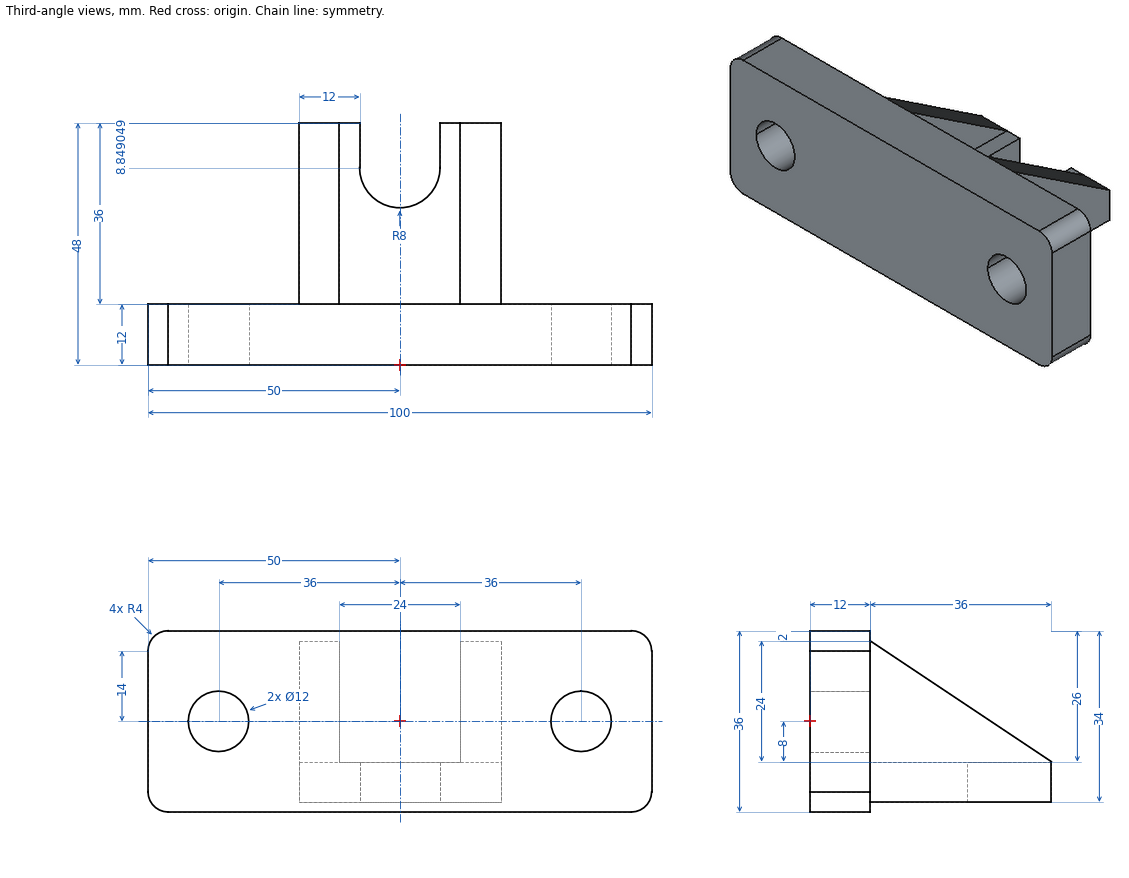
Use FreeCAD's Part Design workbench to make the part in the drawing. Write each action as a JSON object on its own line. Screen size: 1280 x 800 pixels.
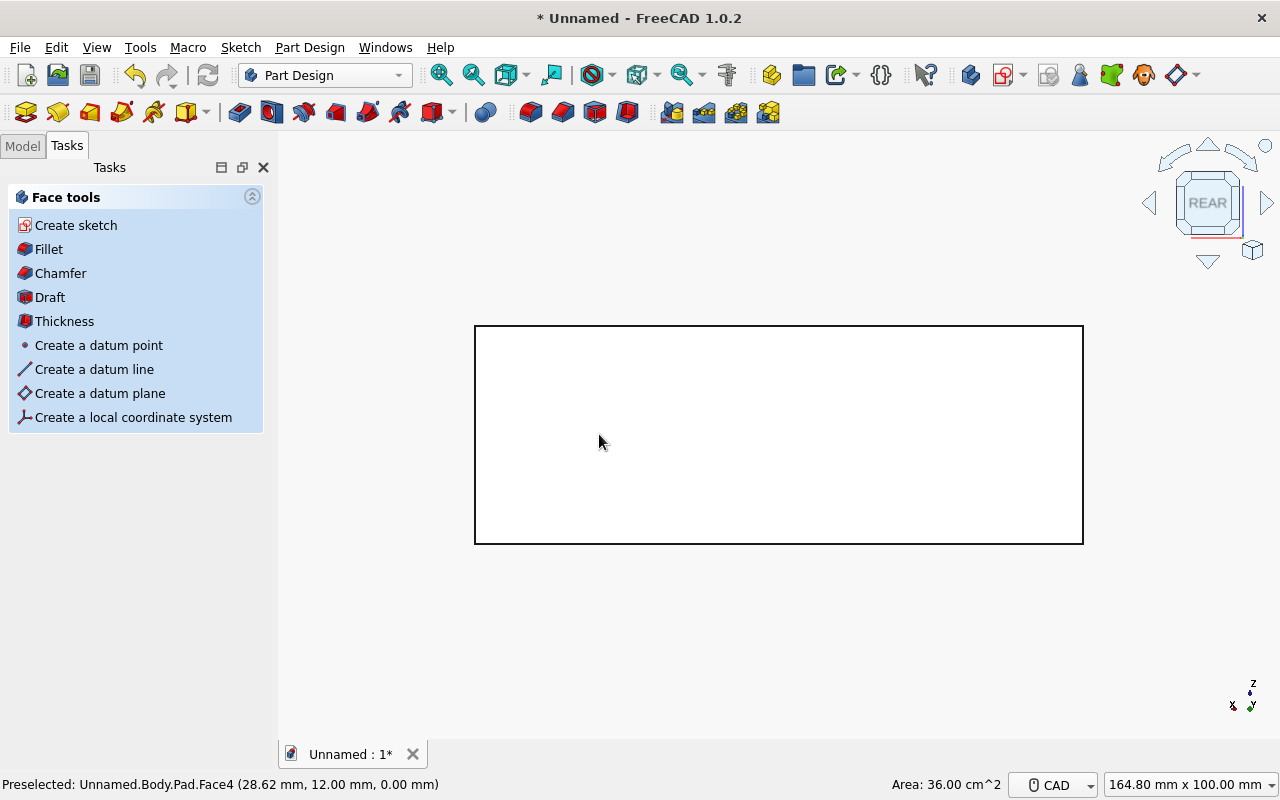
{"action": "left_click", "coordinate": [1004, 76]}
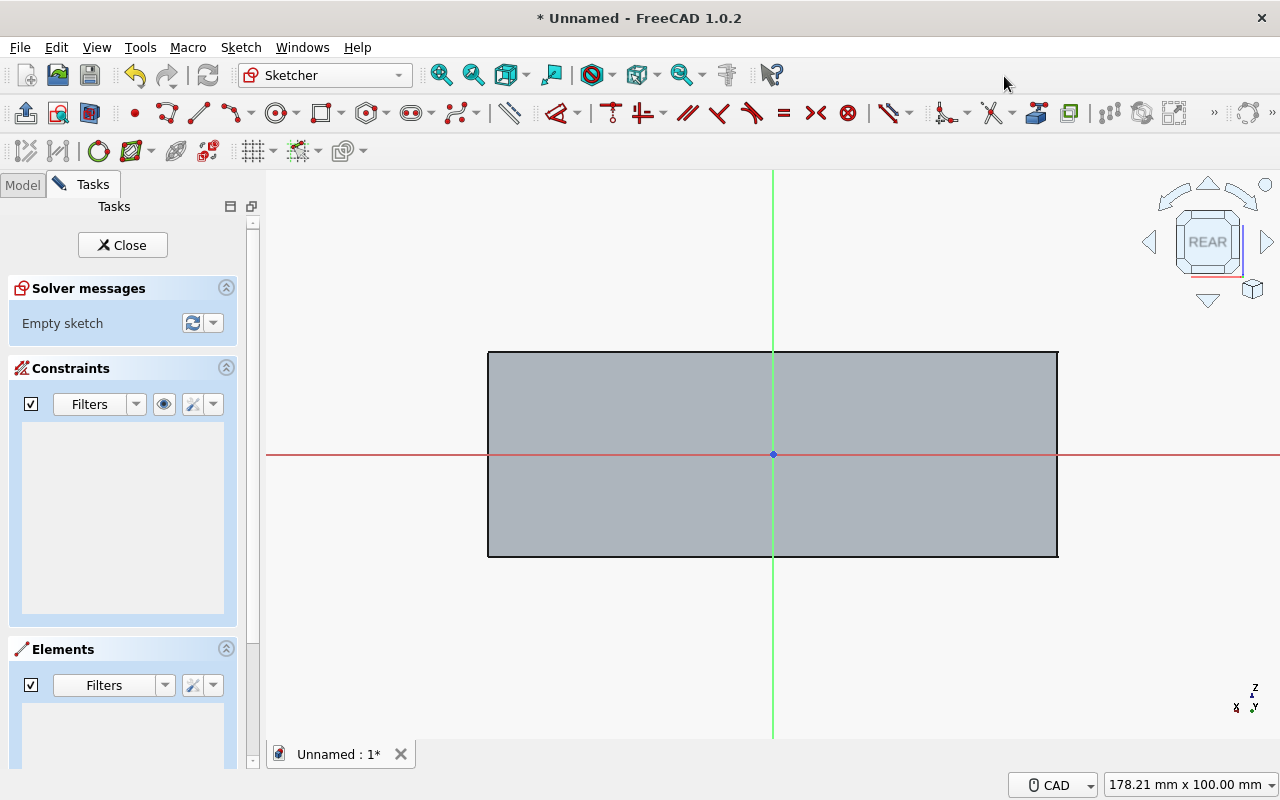
{"action": "left_click", "coordinate": [168, 114]}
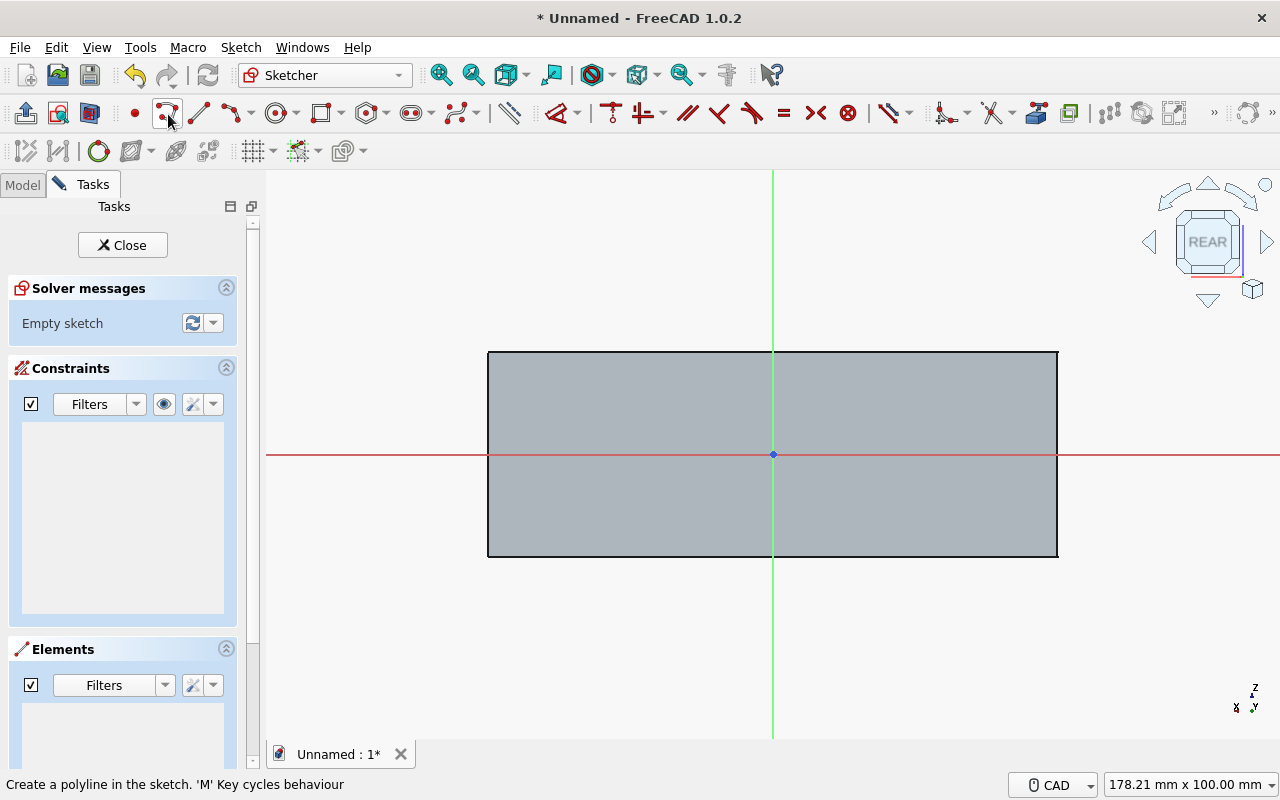
{"action": "left_click", "coordinate": [1058, 375]}
{"action": "left_click", "coordinate": [1058, 352]}
{"action": "left_click", "coordinate": [1035, 352]}
{"action": "right_click", "coordinate": [1035, 352]}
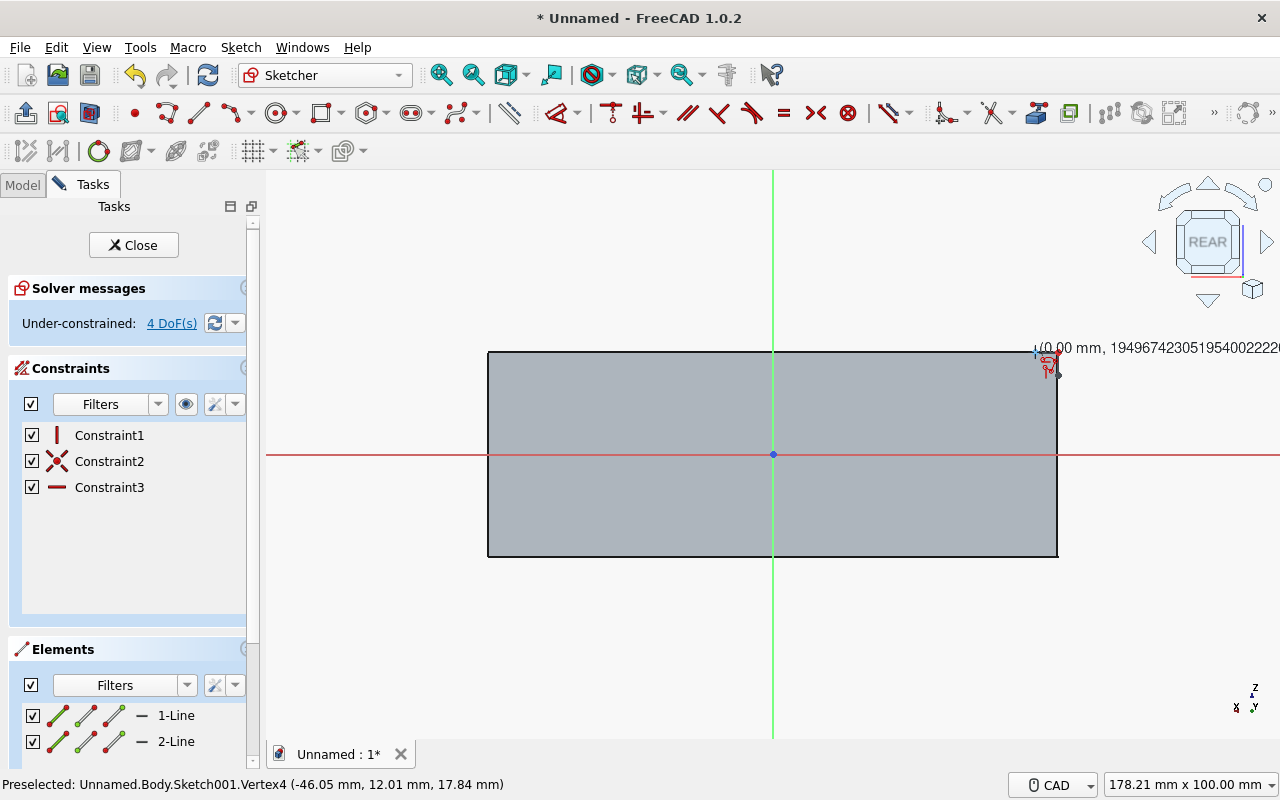
{"action": "left_click", "coordinate": [232, 114]}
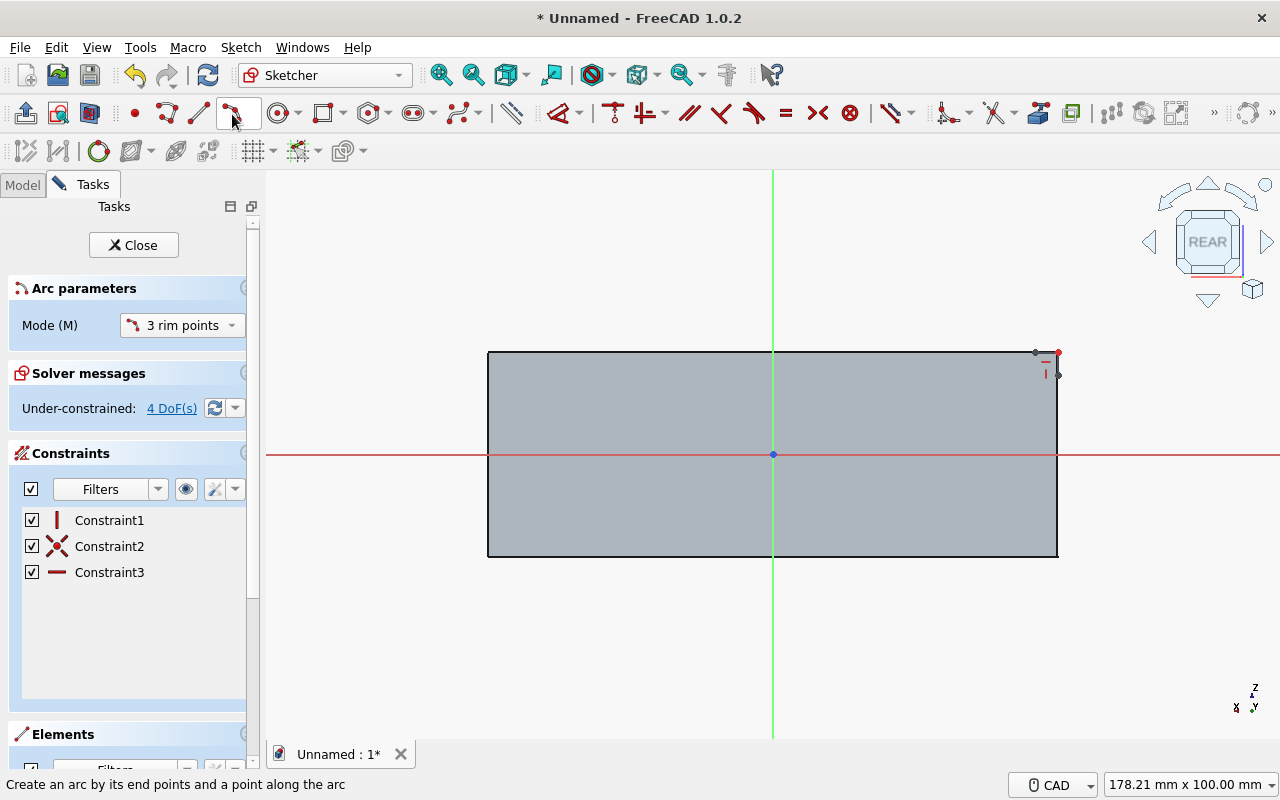
{"action": "scroll", "coordinate": [1035, 352], "scroll_direction": "up", "scroll_amount": 2}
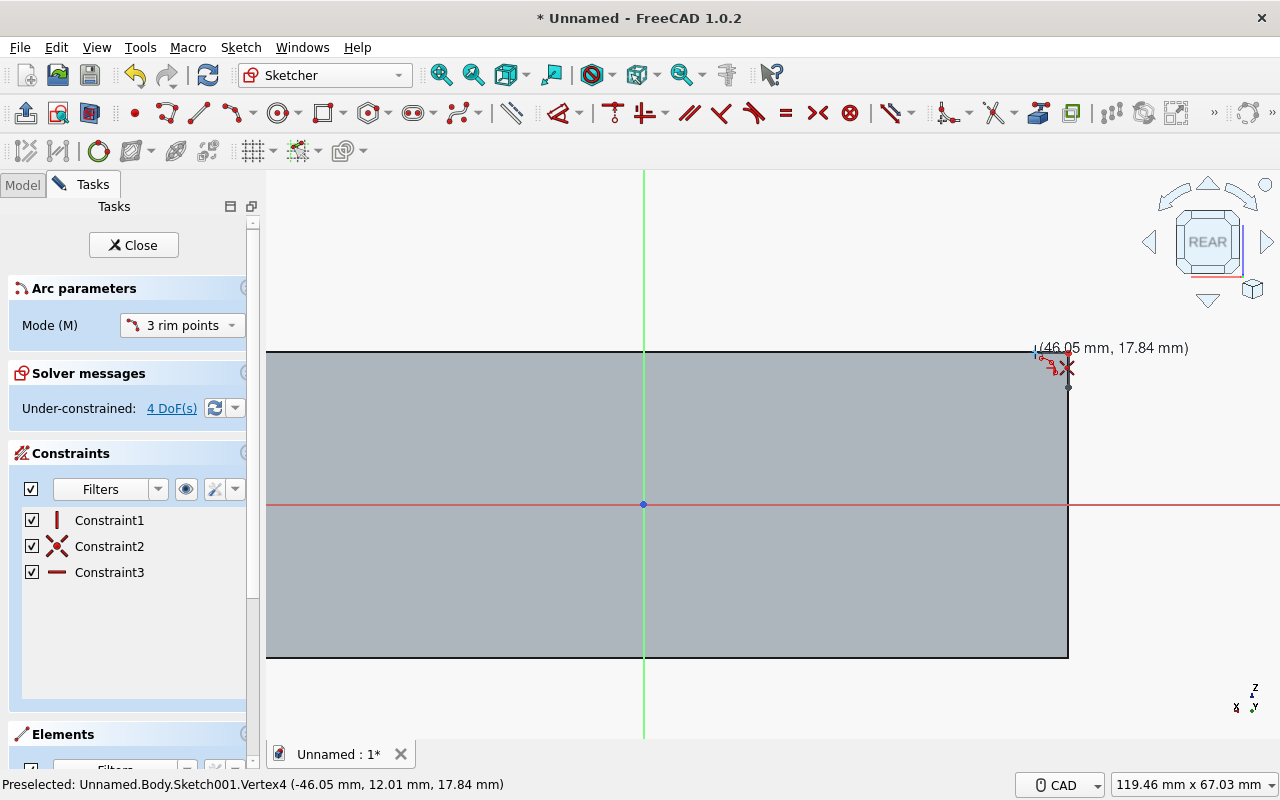
{"action": "left_click", "coordinate": [1035, 353]}
{"action": "left_click", "coordinate": [1069, 388]}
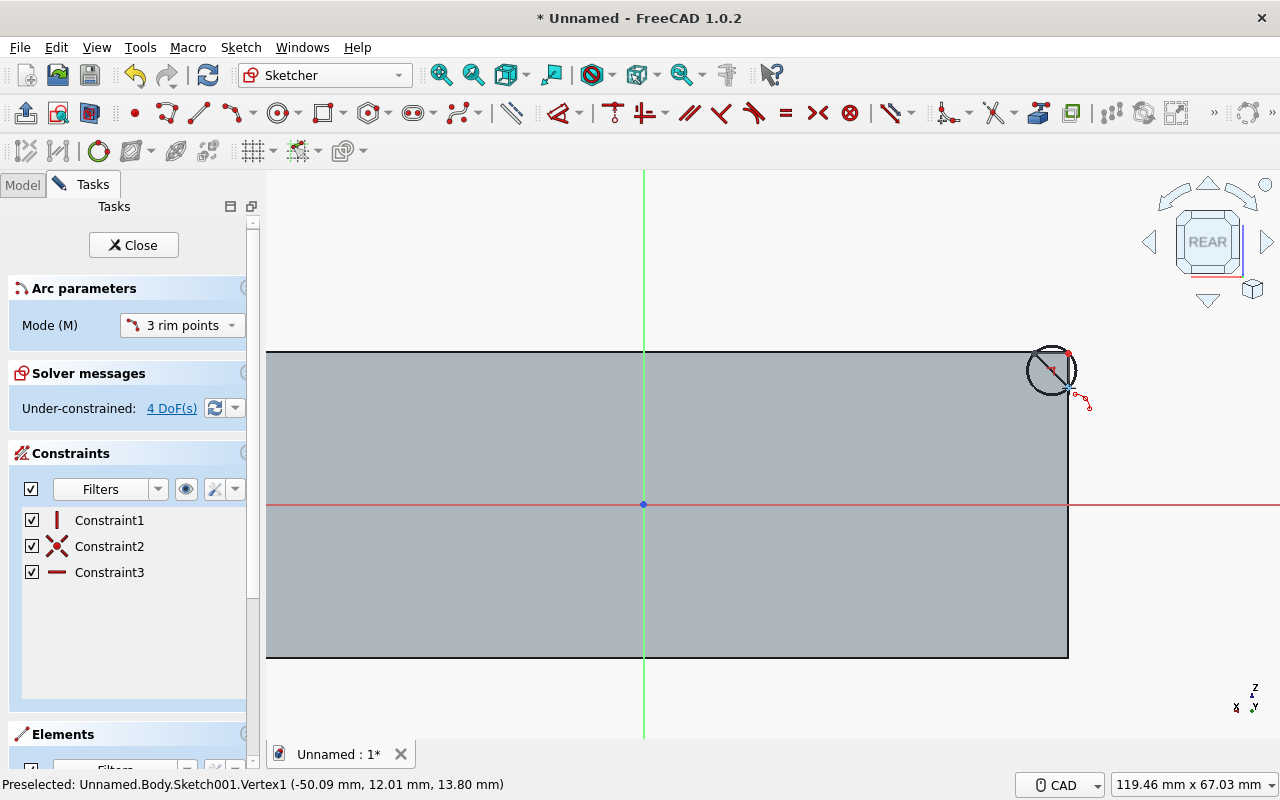
{"action": "scroll", "coordinate": [1058, 362], "scroll_direction": "up", "scroll_amount": 3}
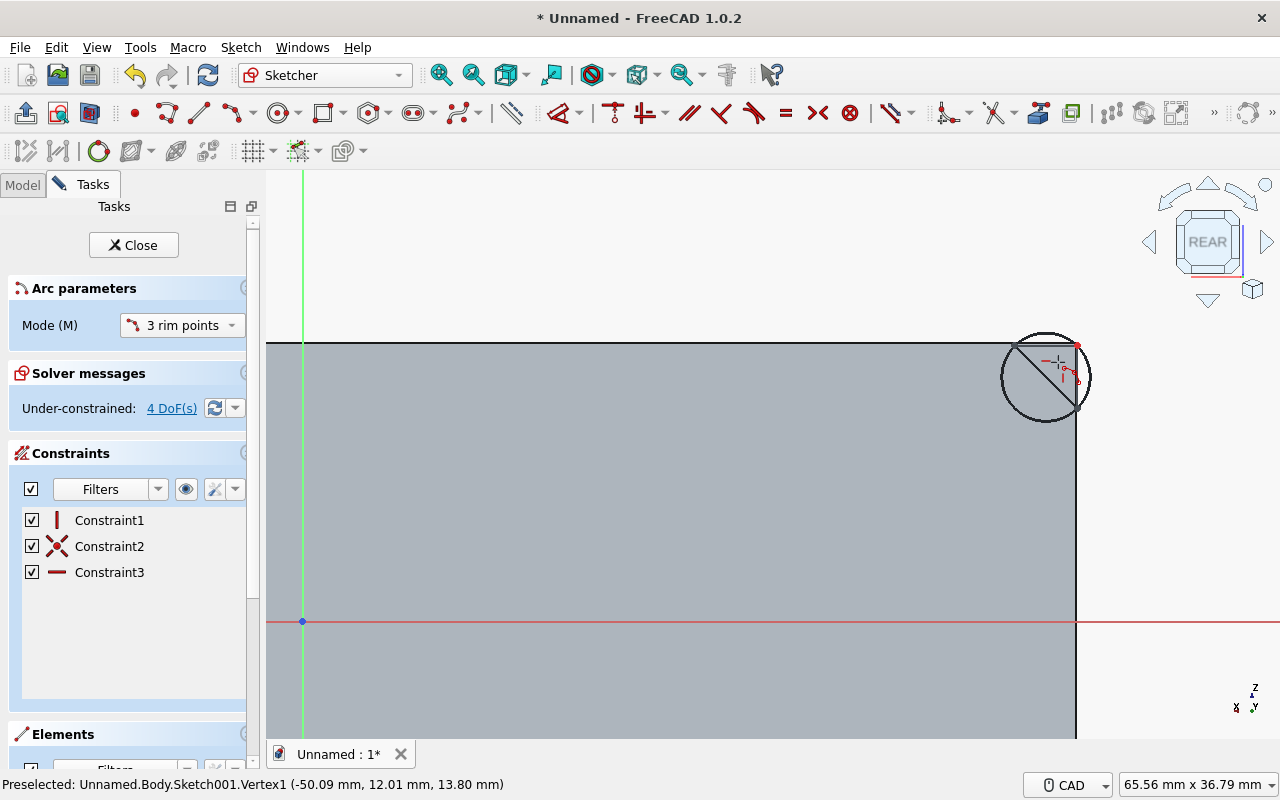
{"action": "left_click", "coordinate": [1058, 362]}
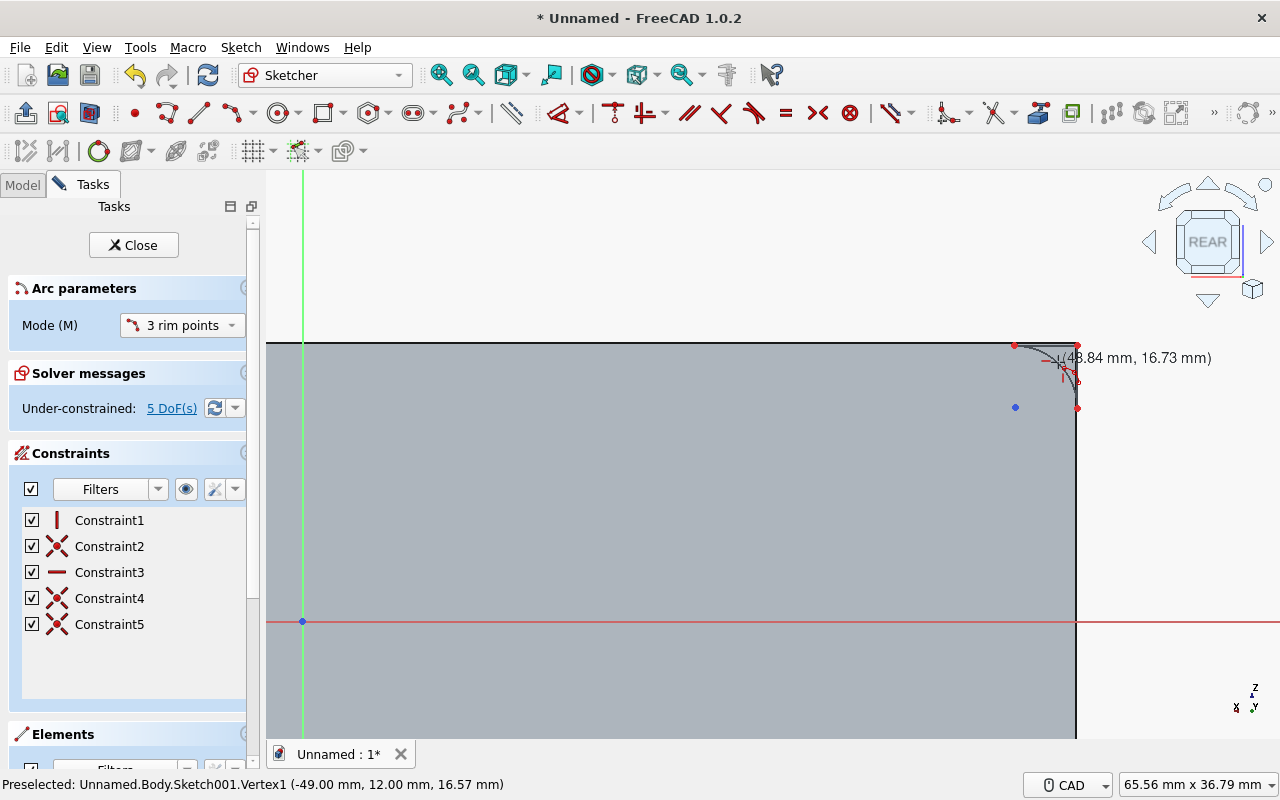
{"action": "left_click", "coordinate": [168, 114]}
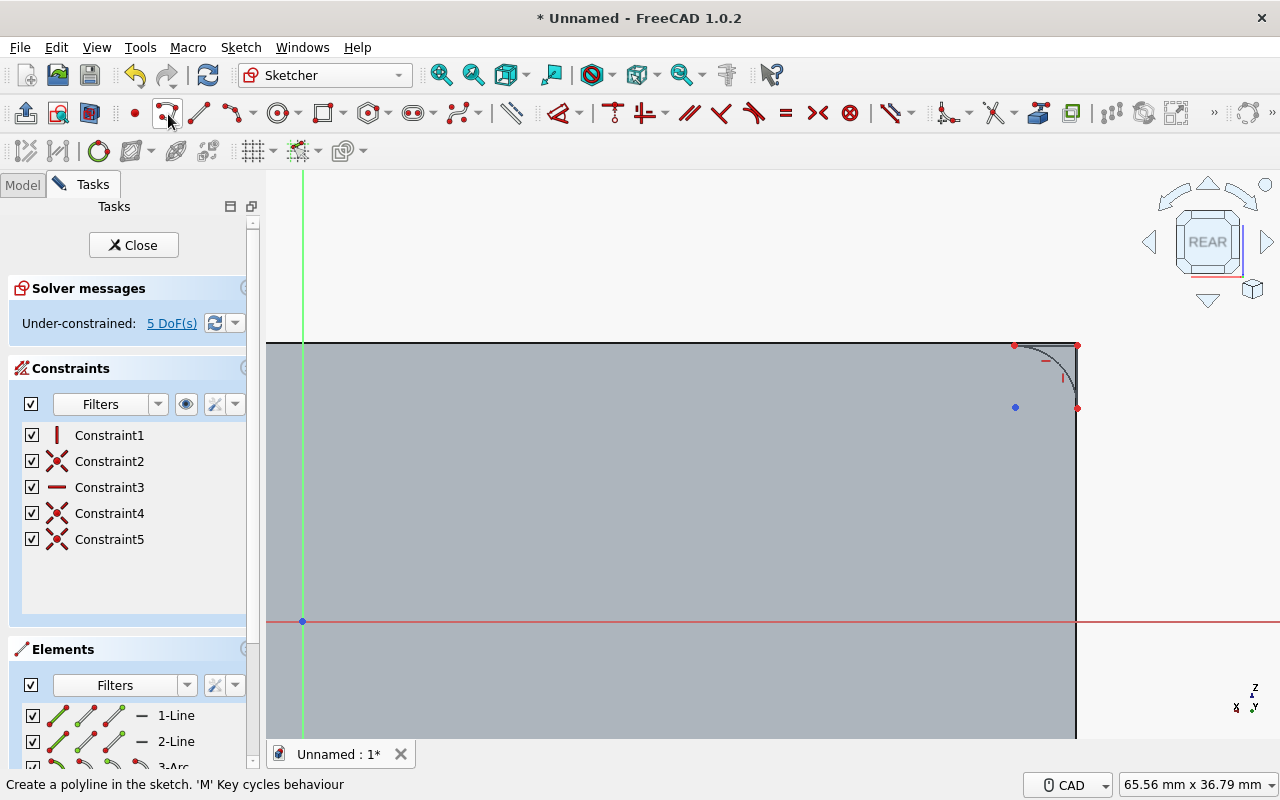
{"action": "scroll", "coordinate": [938, 357], "scroll_direction": "down", "scroll_amount": 5}